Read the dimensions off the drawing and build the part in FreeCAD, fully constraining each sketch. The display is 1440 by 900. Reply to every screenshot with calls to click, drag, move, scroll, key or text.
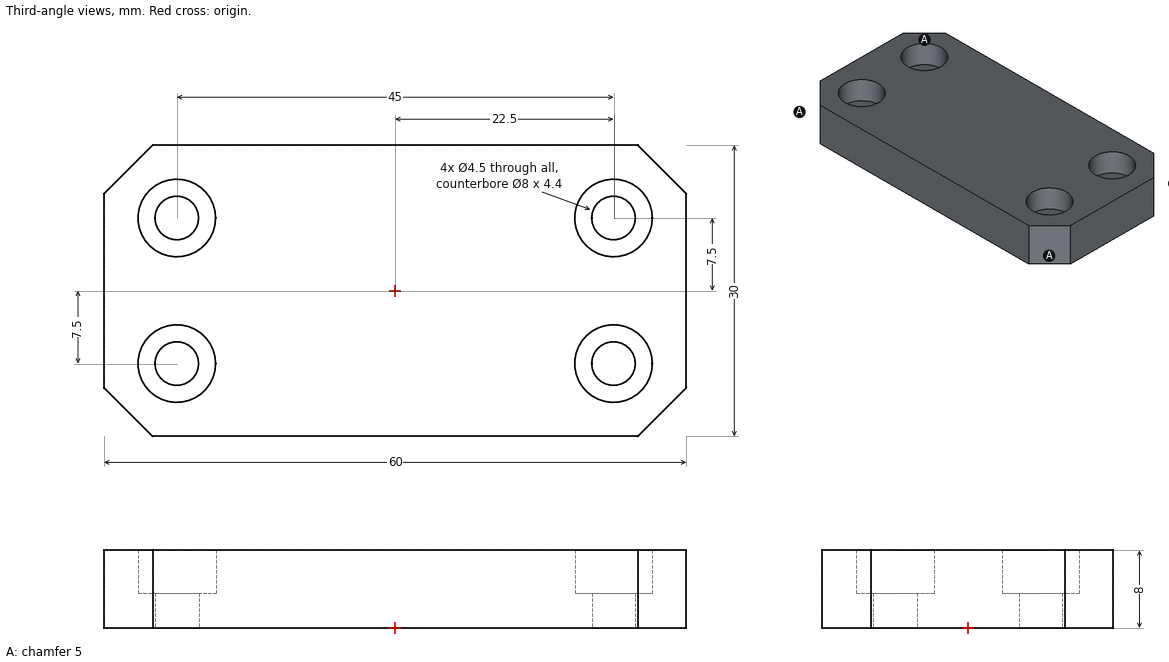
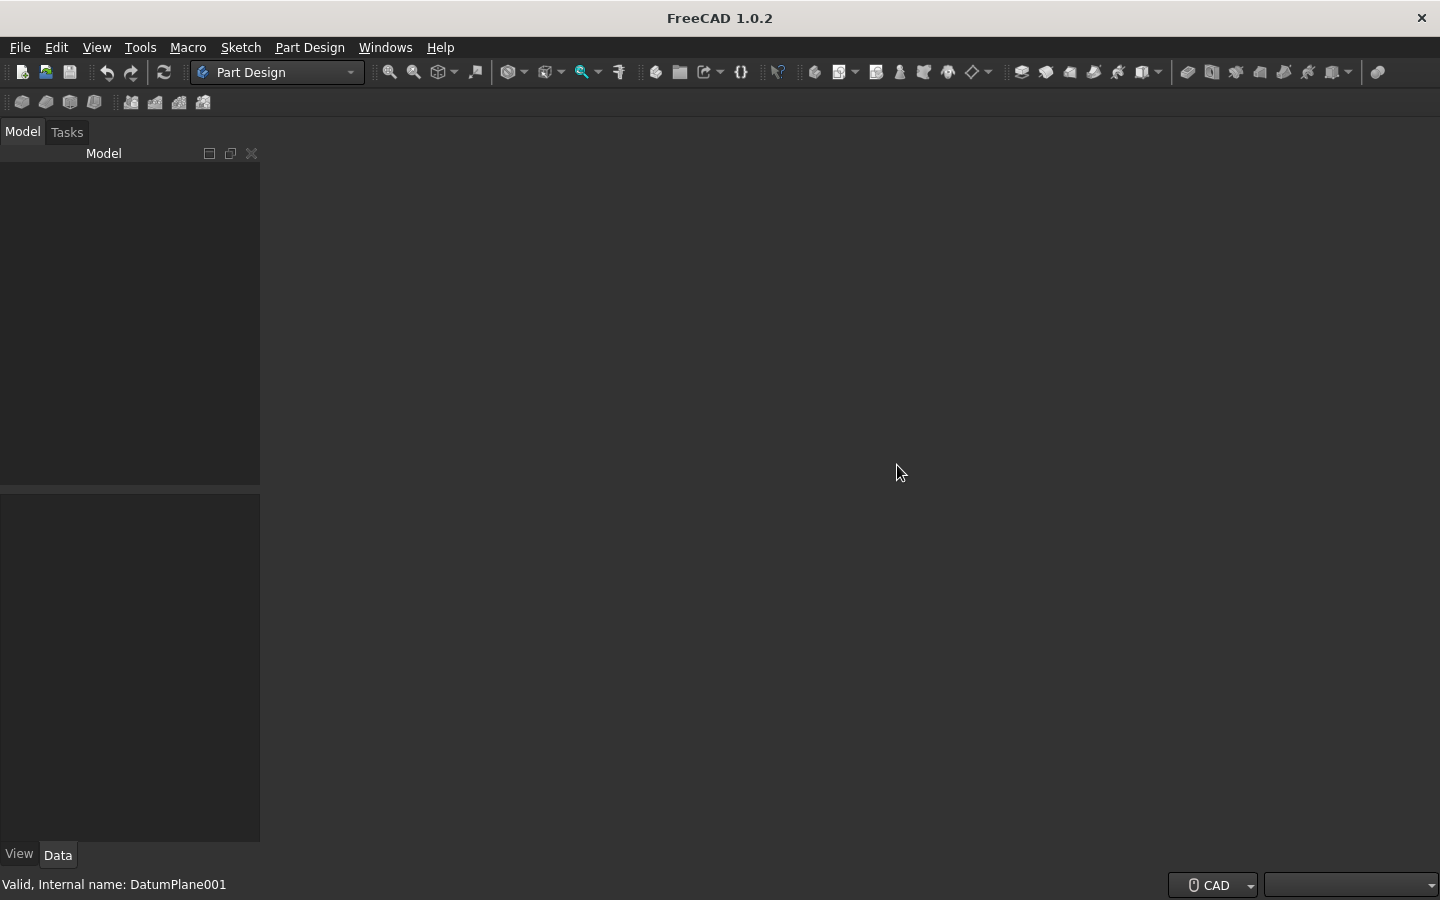
click(22, 72)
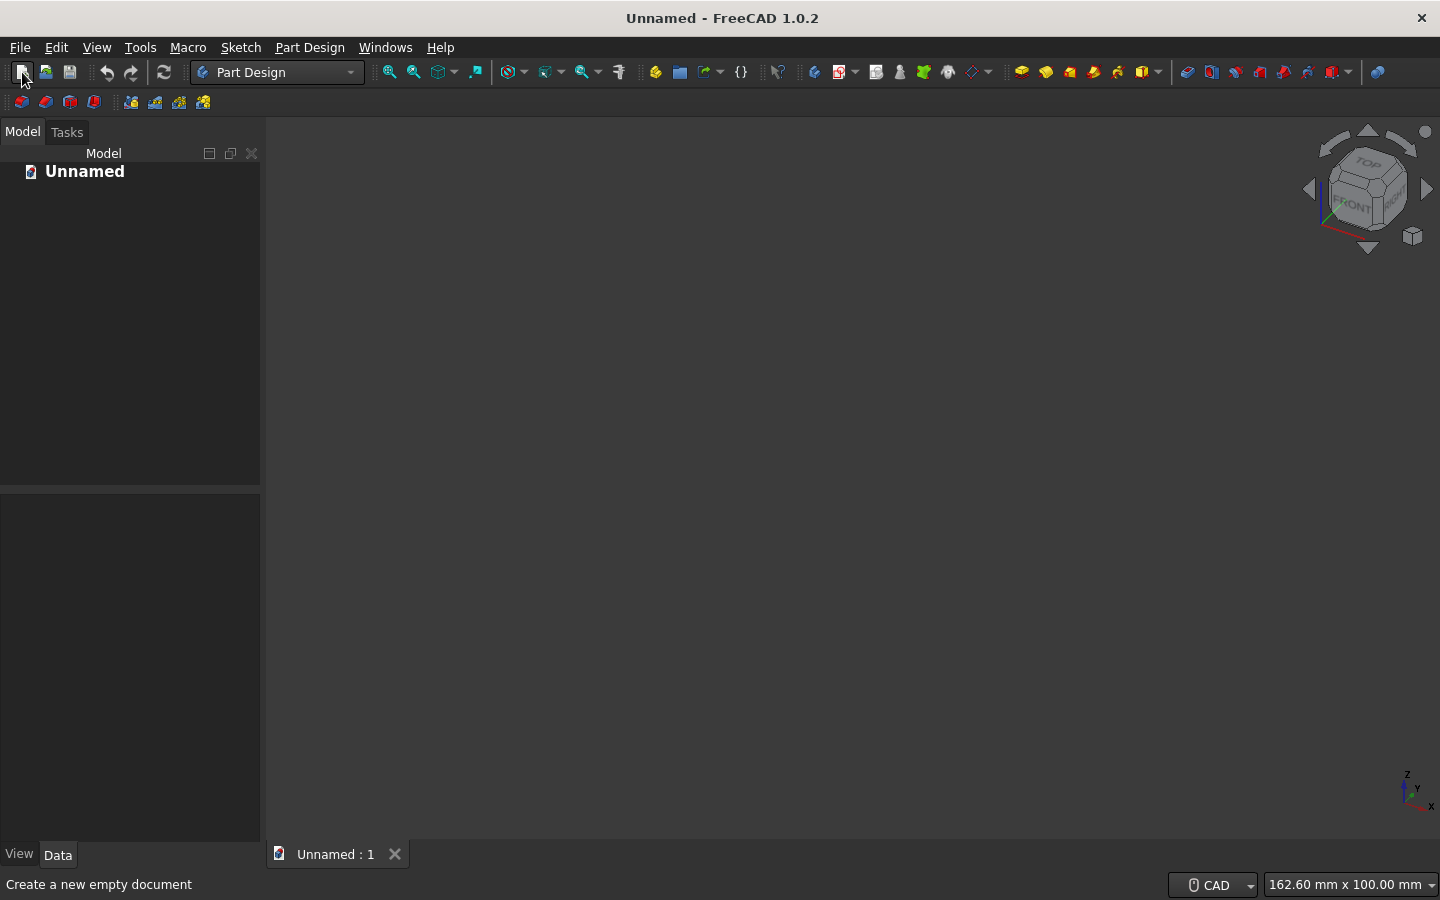
click(840, 72)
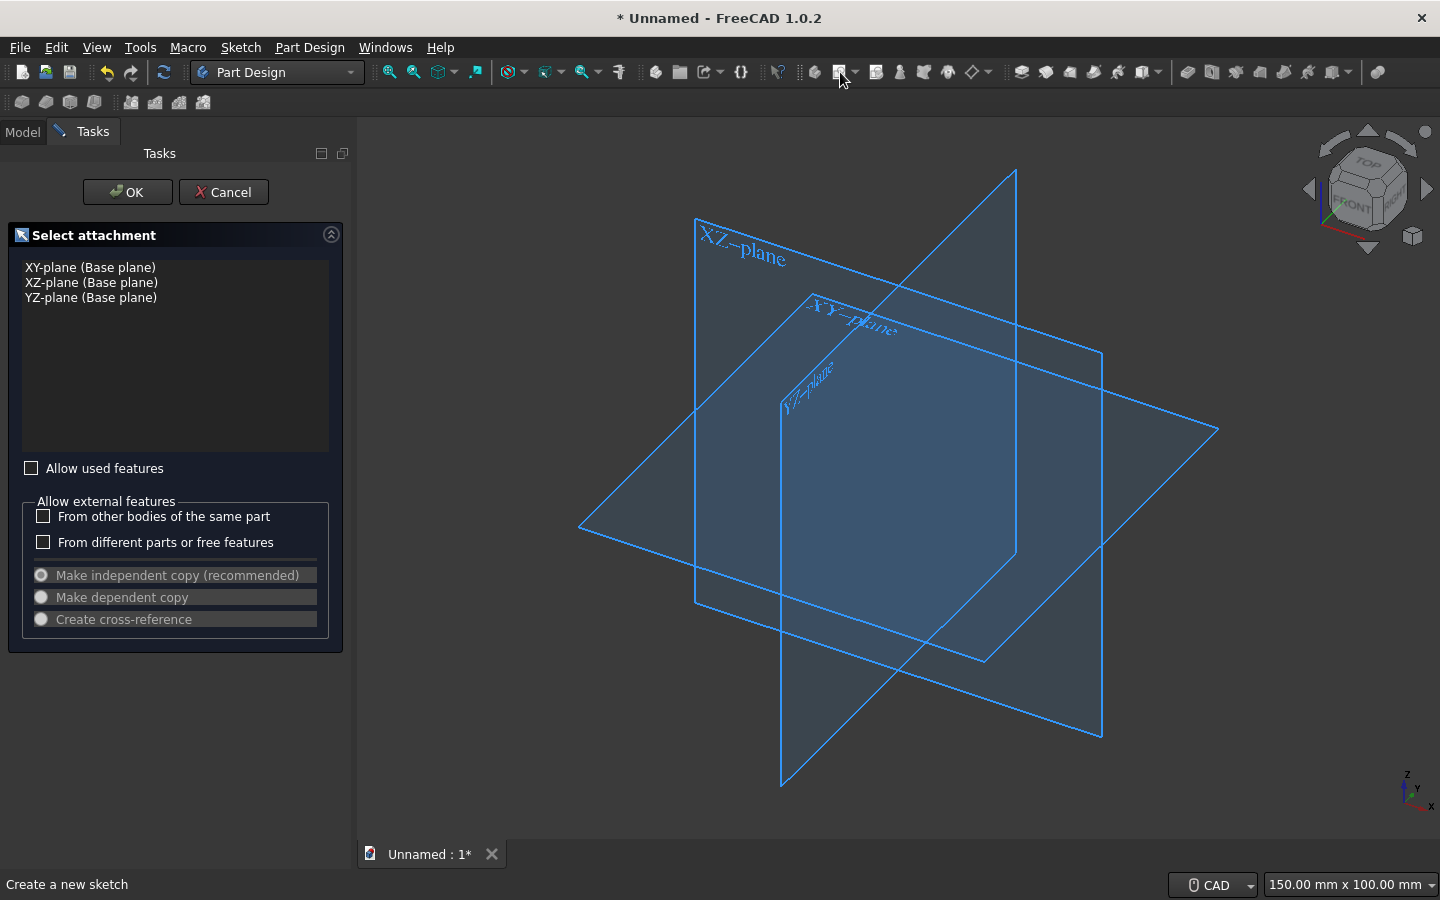
click(82, 268)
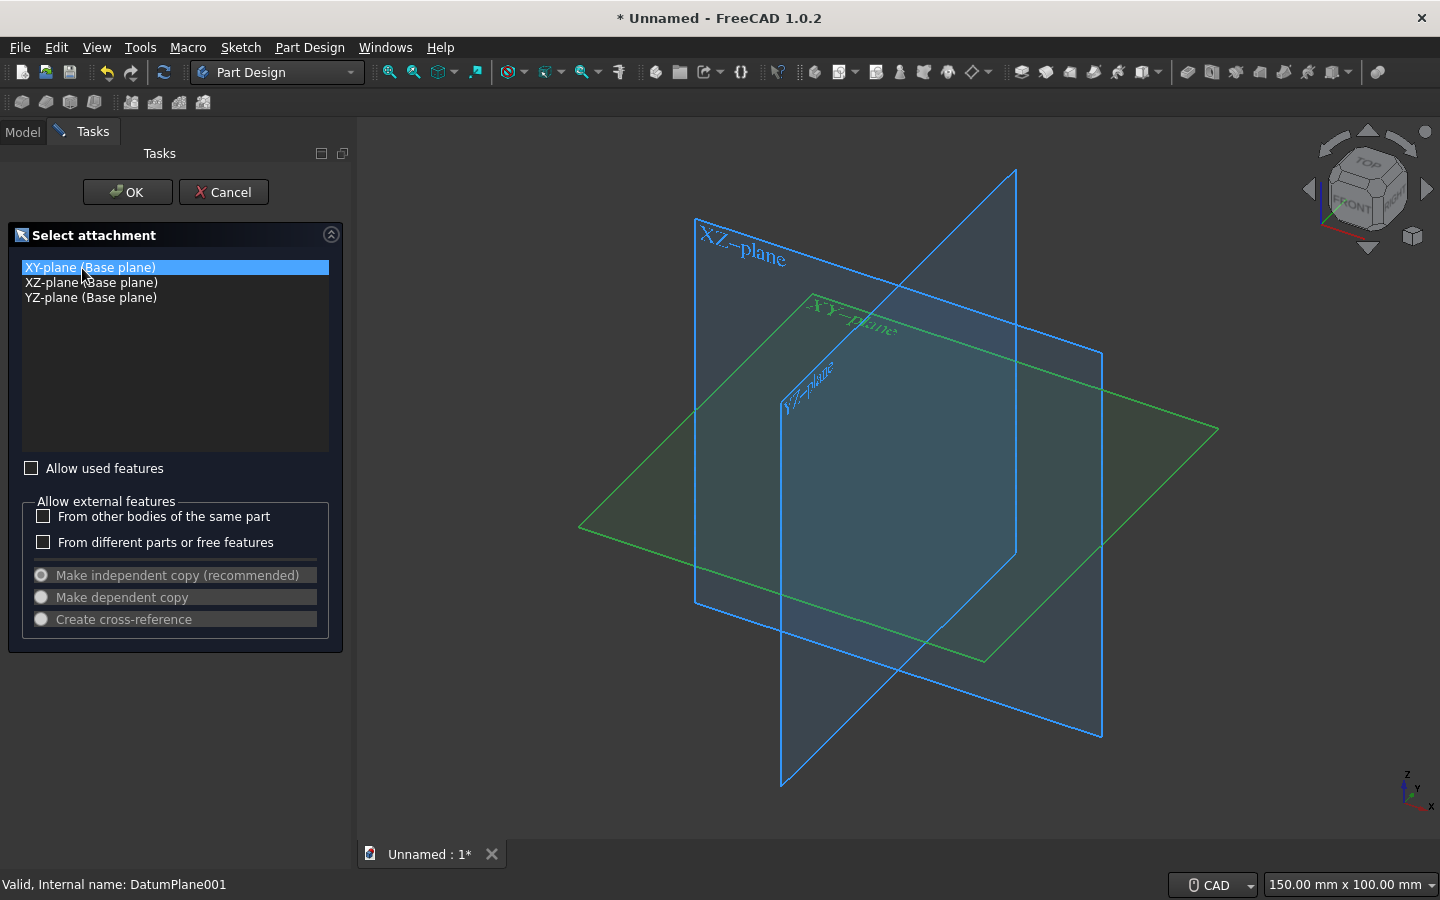
click(128, 192)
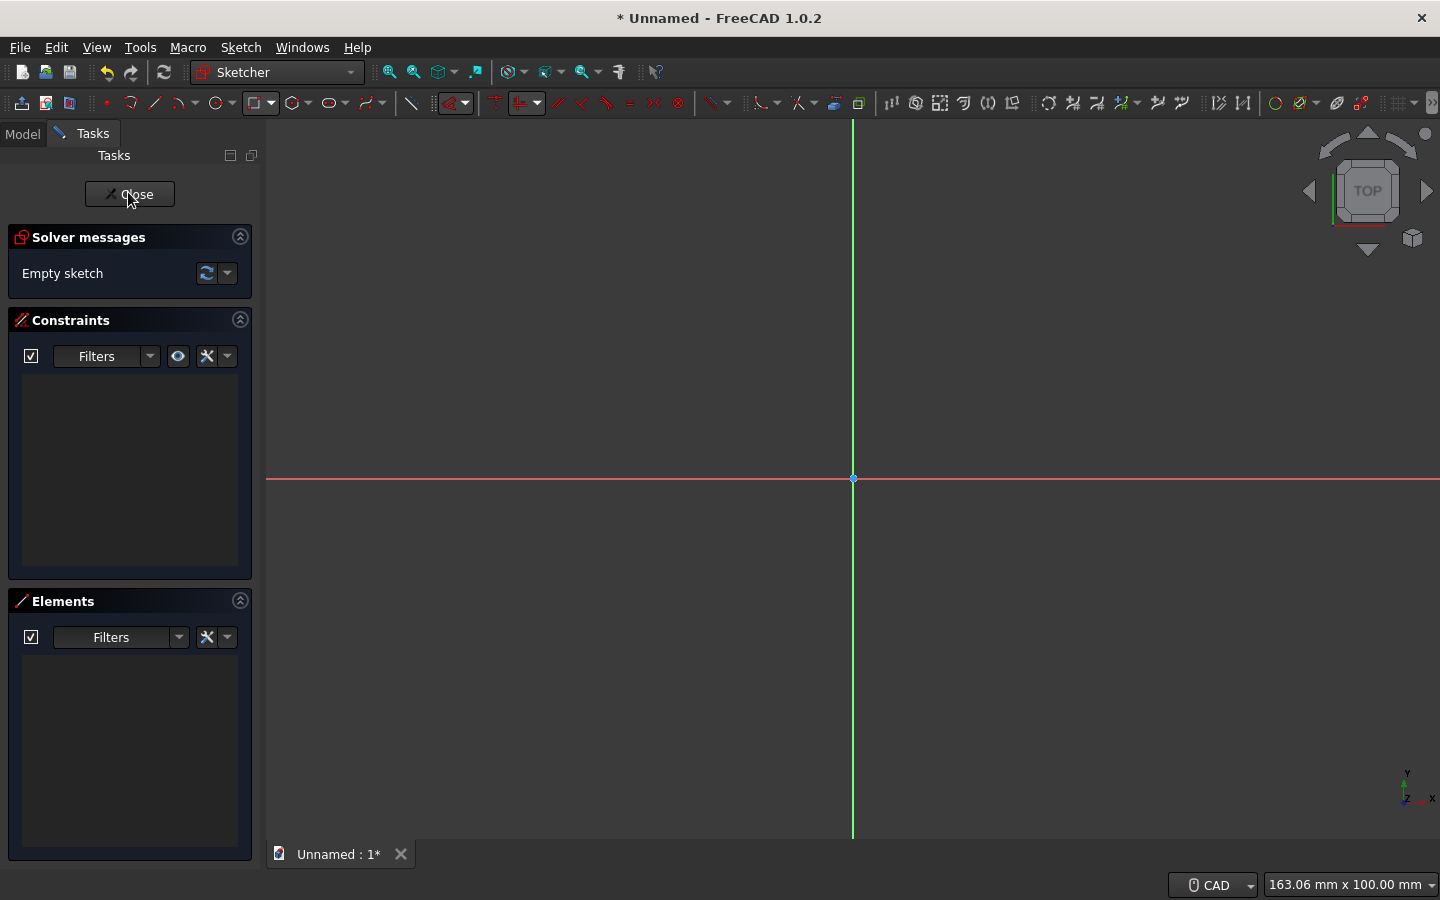
scroll(992, 479, up, 2)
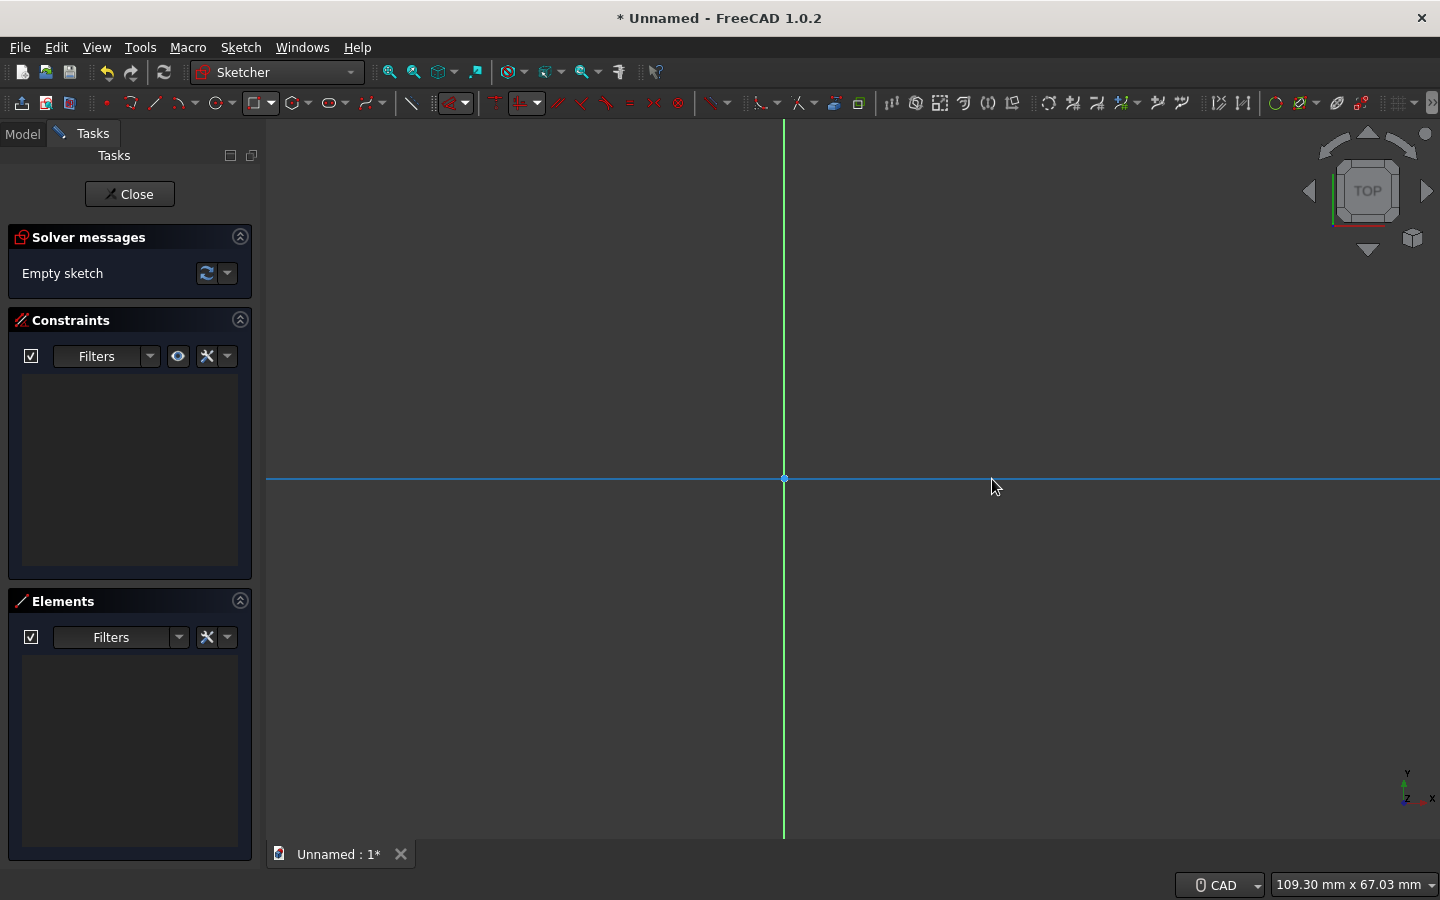
click(274, 104)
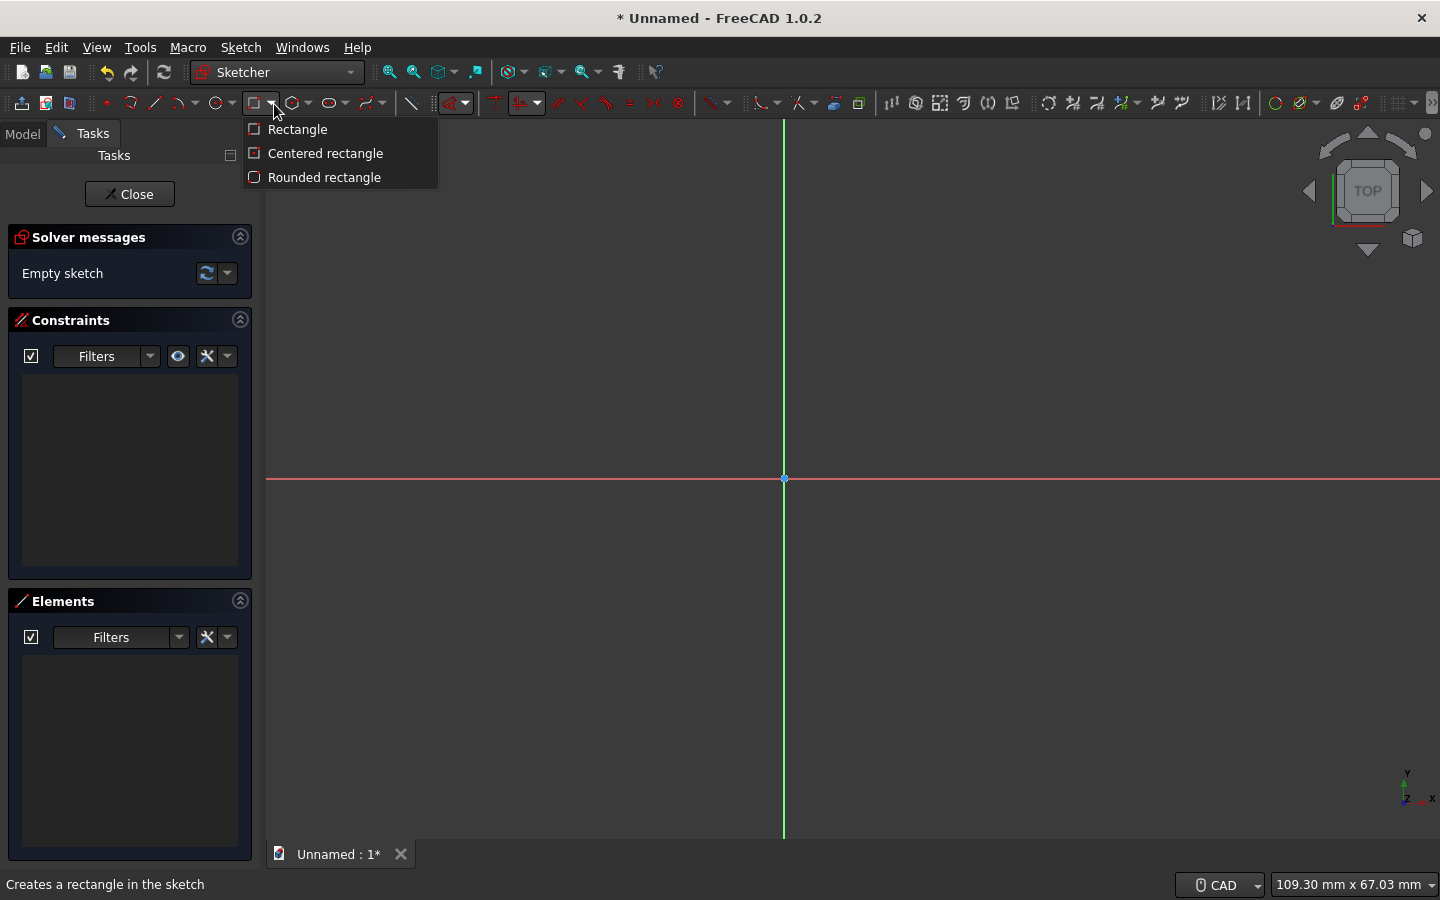
click(340, 153)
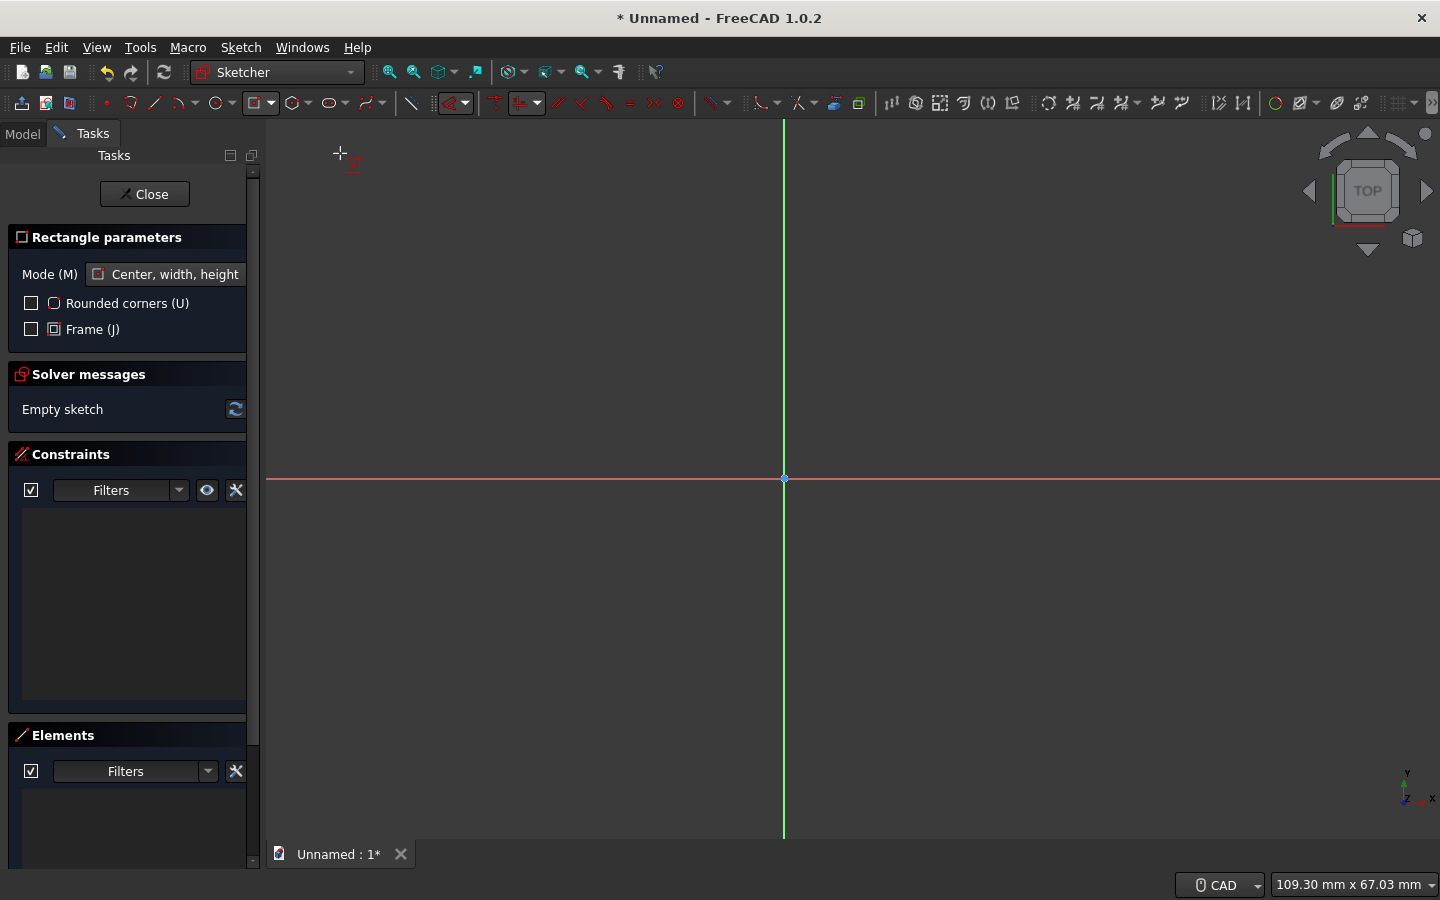
click(784, 479)
click(1107, 318)
key(Escape)